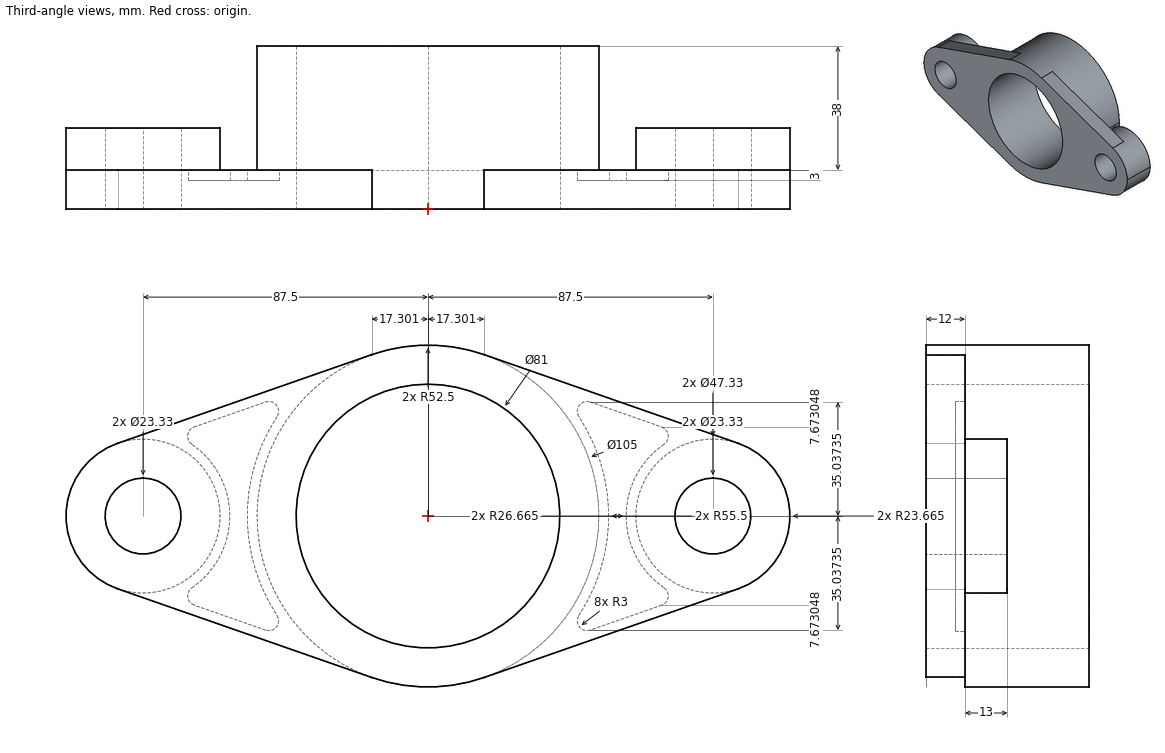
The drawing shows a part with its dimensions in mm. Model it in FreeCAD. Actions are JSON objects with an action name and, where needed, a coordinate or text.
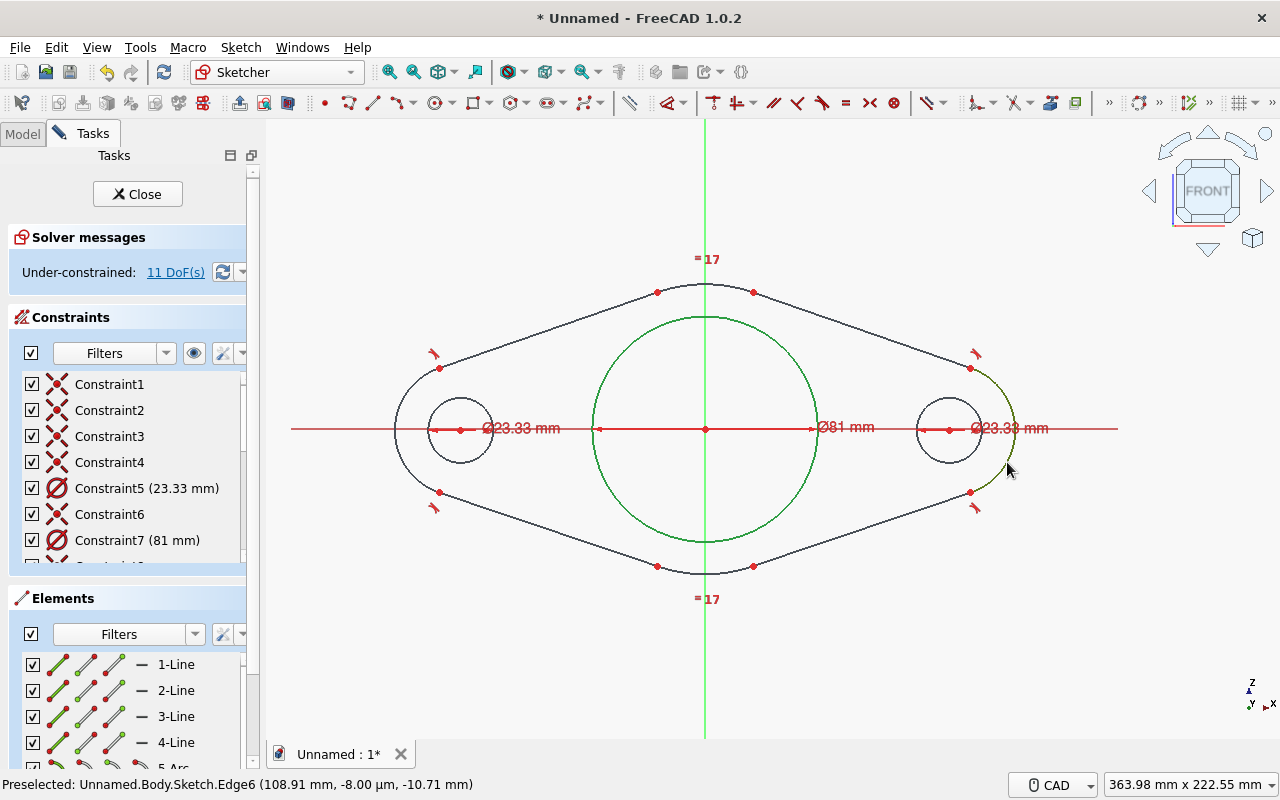
{"action": "left_click", "coordinate": [403, 399]}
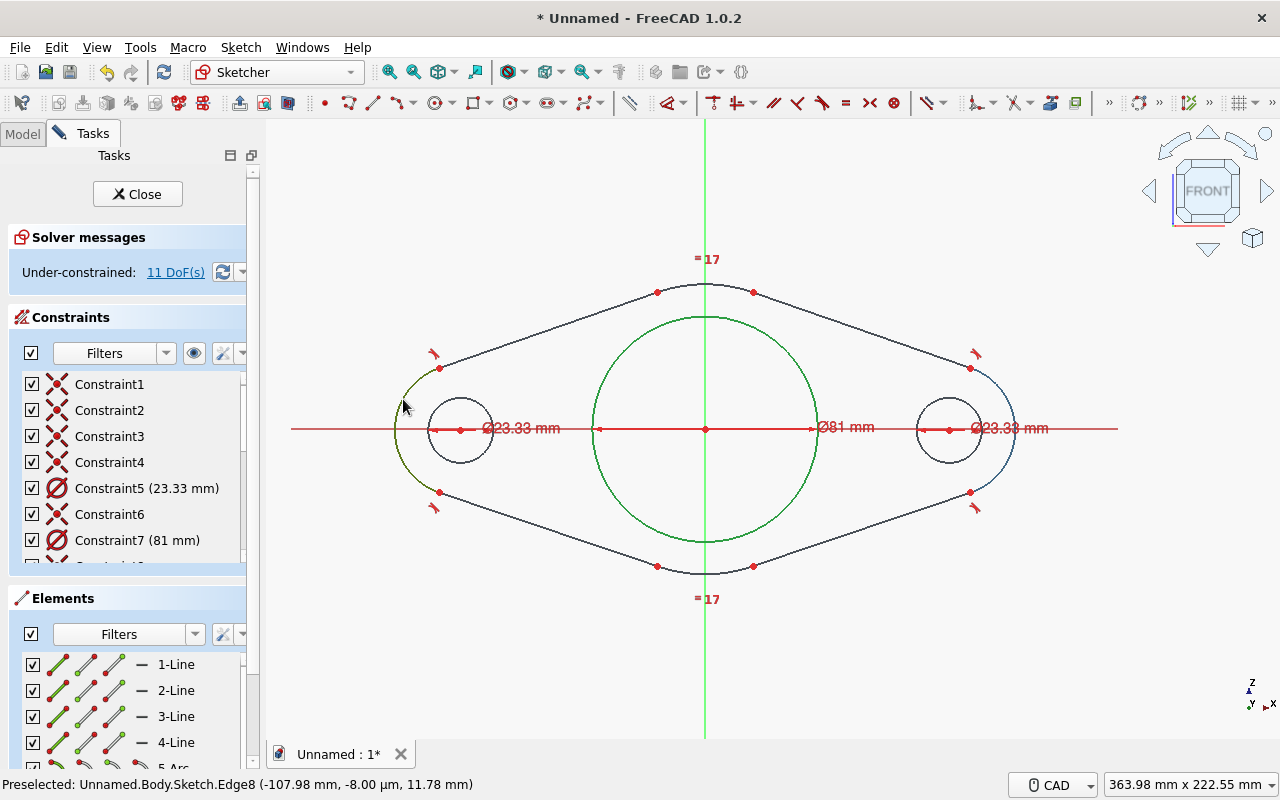
{"action": "left_click", "coordinate": [846, 104]}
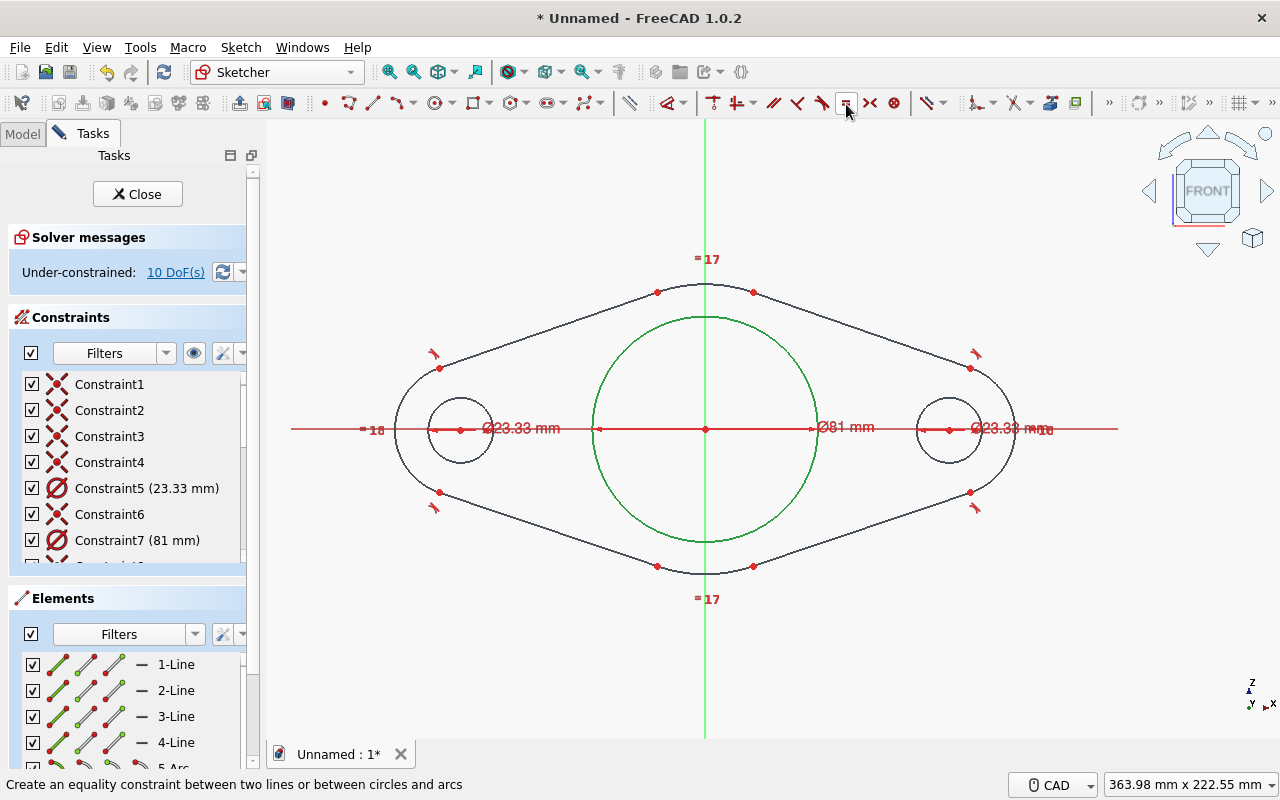
{"action": "left_click", "coordinate": [949, 430]}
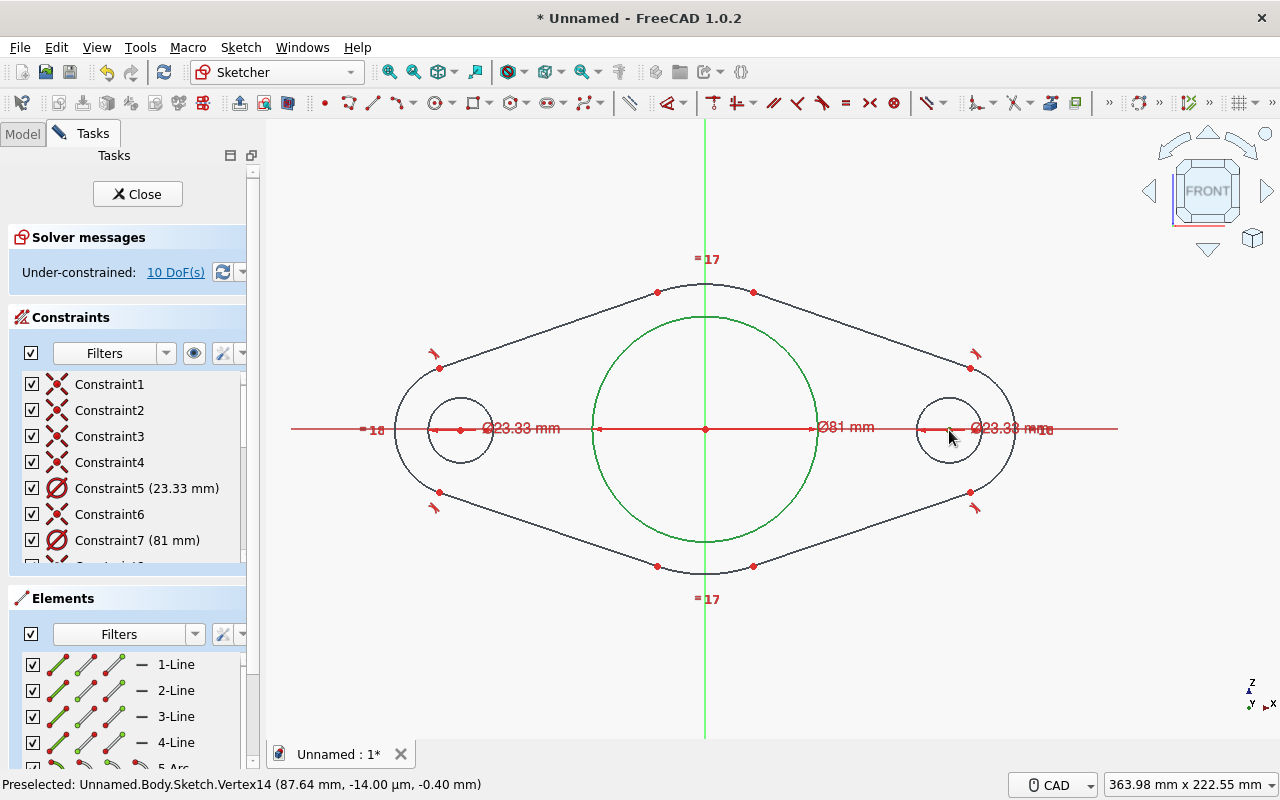
{"action": "left_click", "coordinate": [353, 429]}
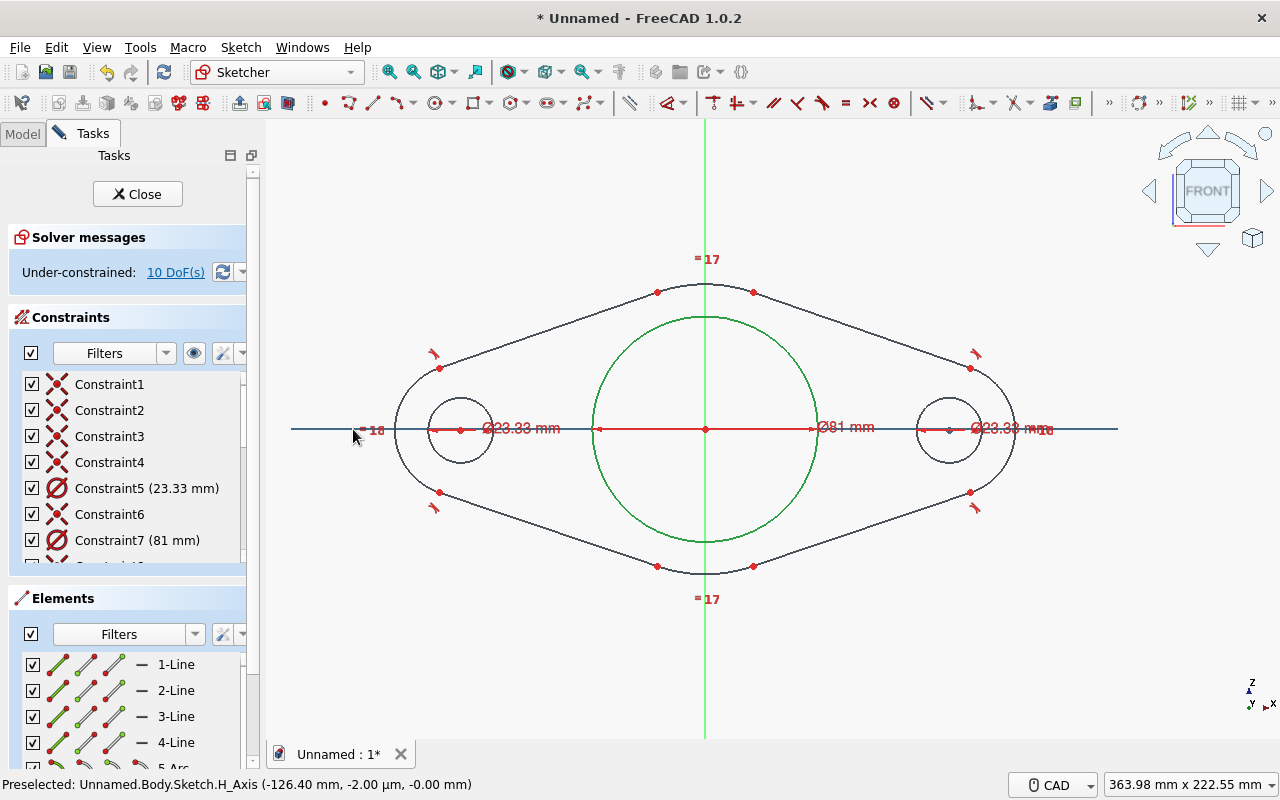
{"action": "left_click", "coordinate": [714, 104]}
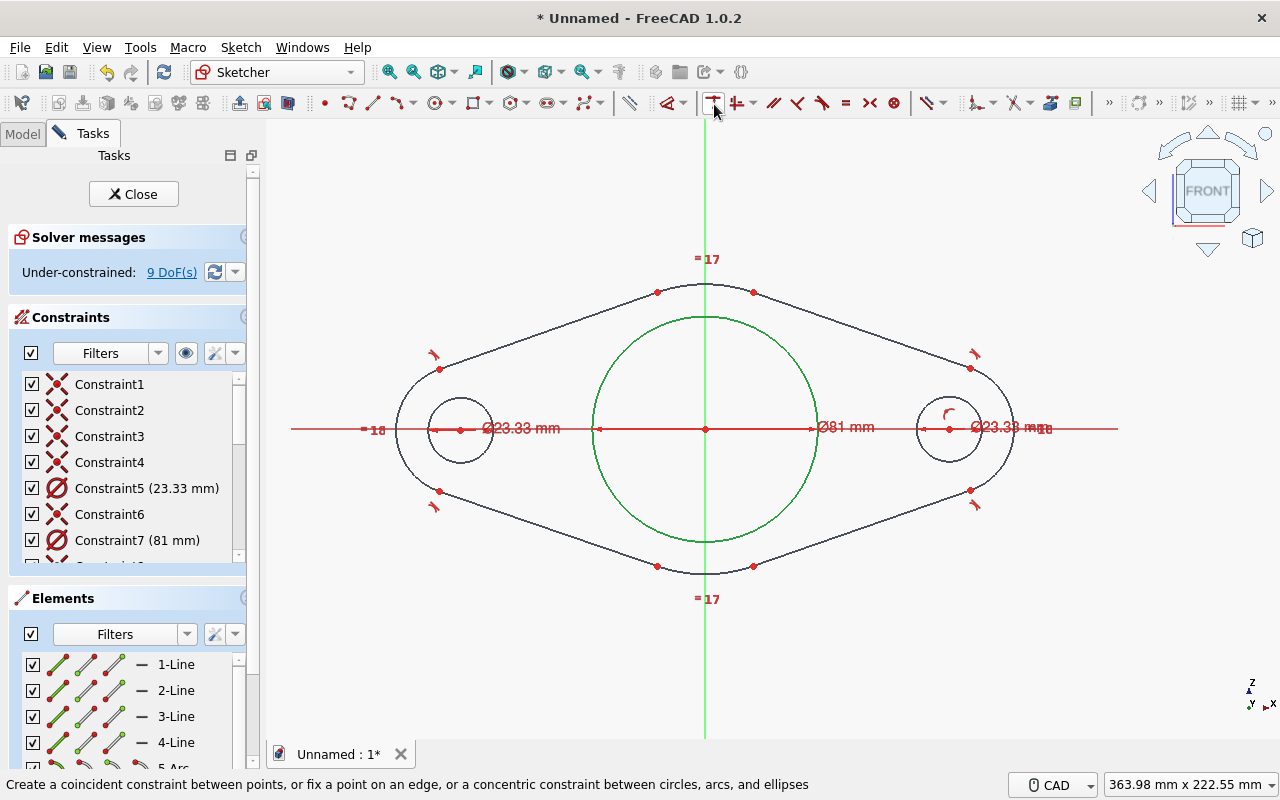
{"action": "left_click", "coordinate": [461, 430]}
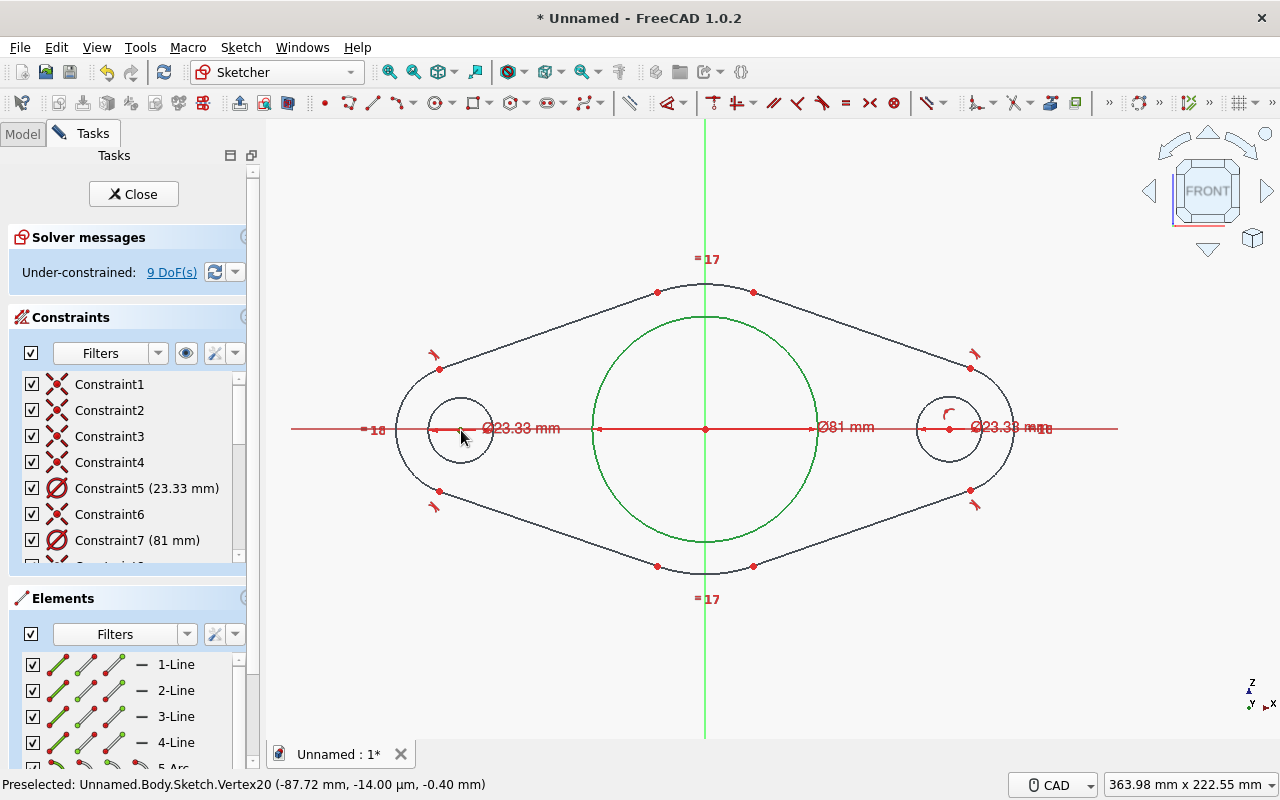
{"action": "left_click", "coordinate": [353, 429]}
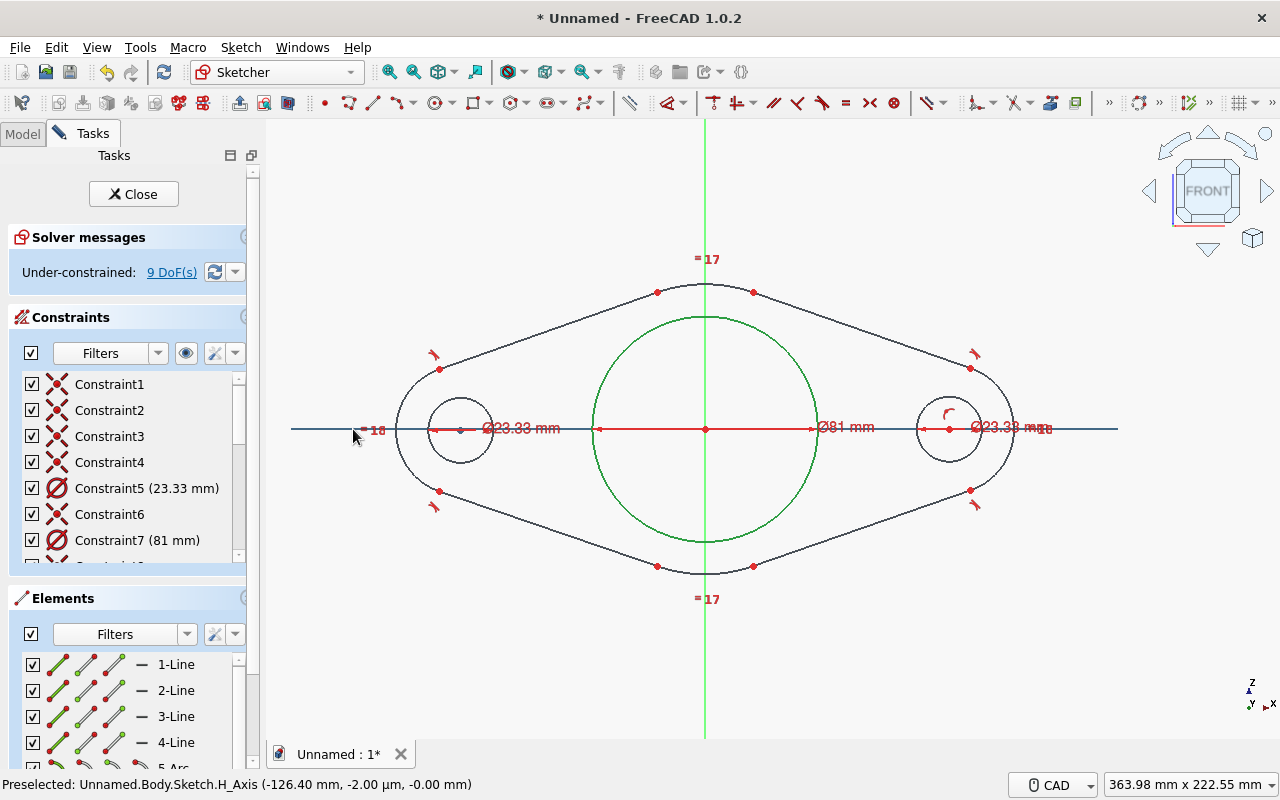
{"action": "left_click", "coordinate": [714, 104]}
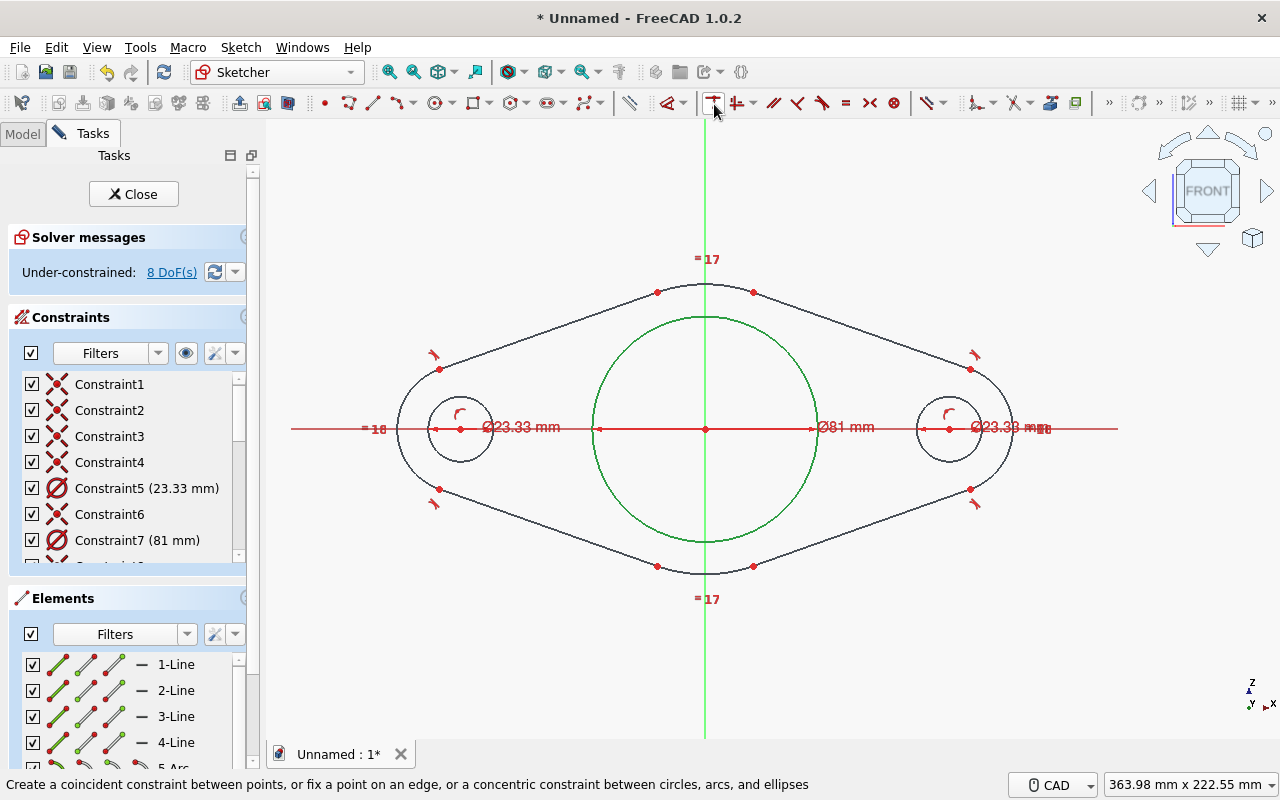
{"action": "left_click", "coordinate": [725, 286]}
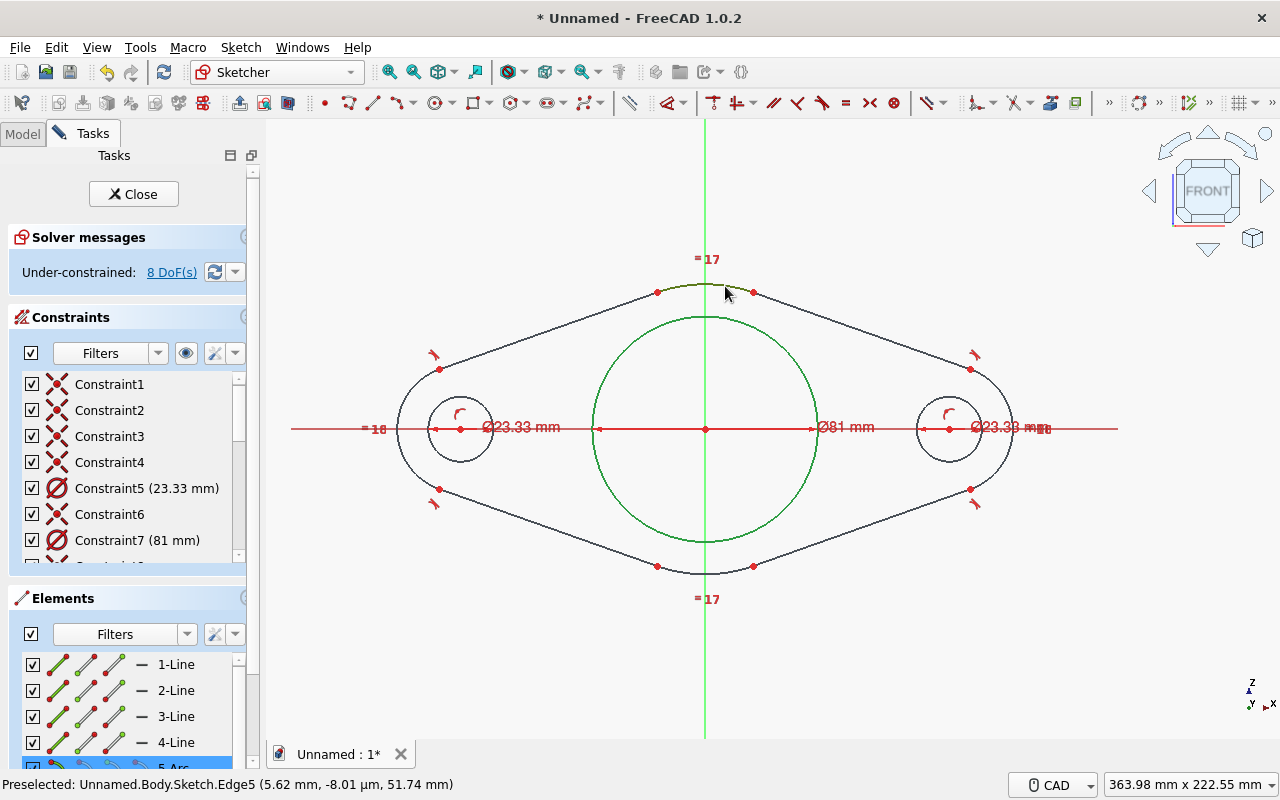
{"action": "key", "text": "k r"}